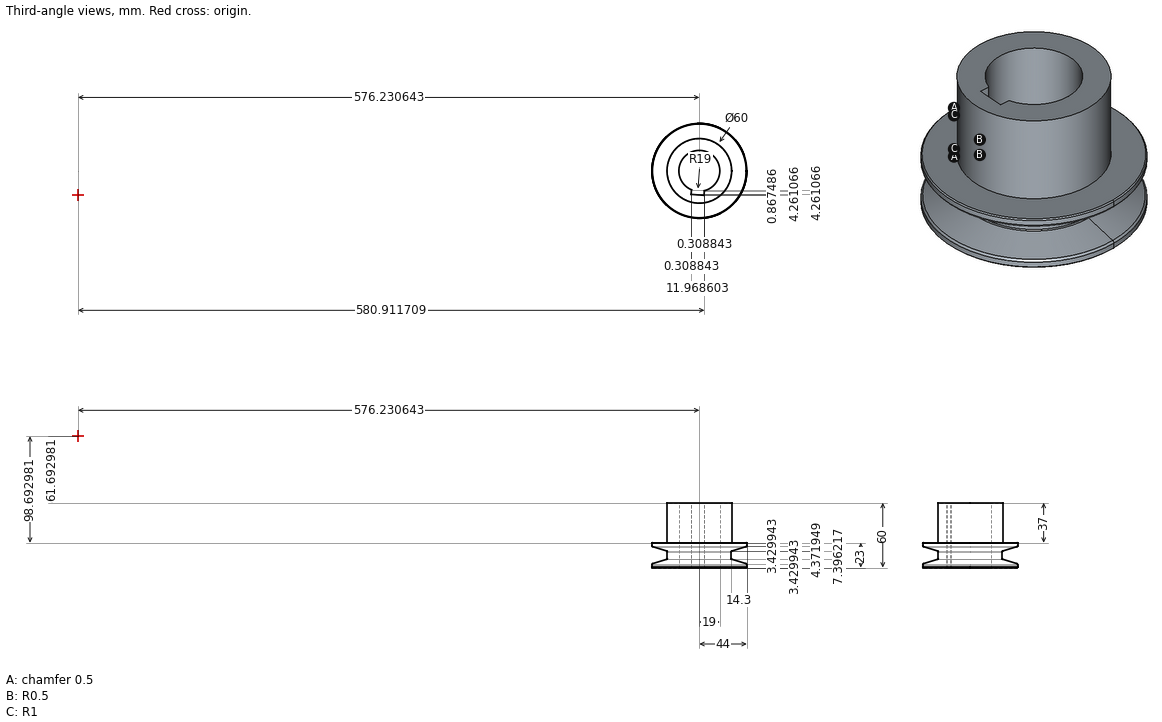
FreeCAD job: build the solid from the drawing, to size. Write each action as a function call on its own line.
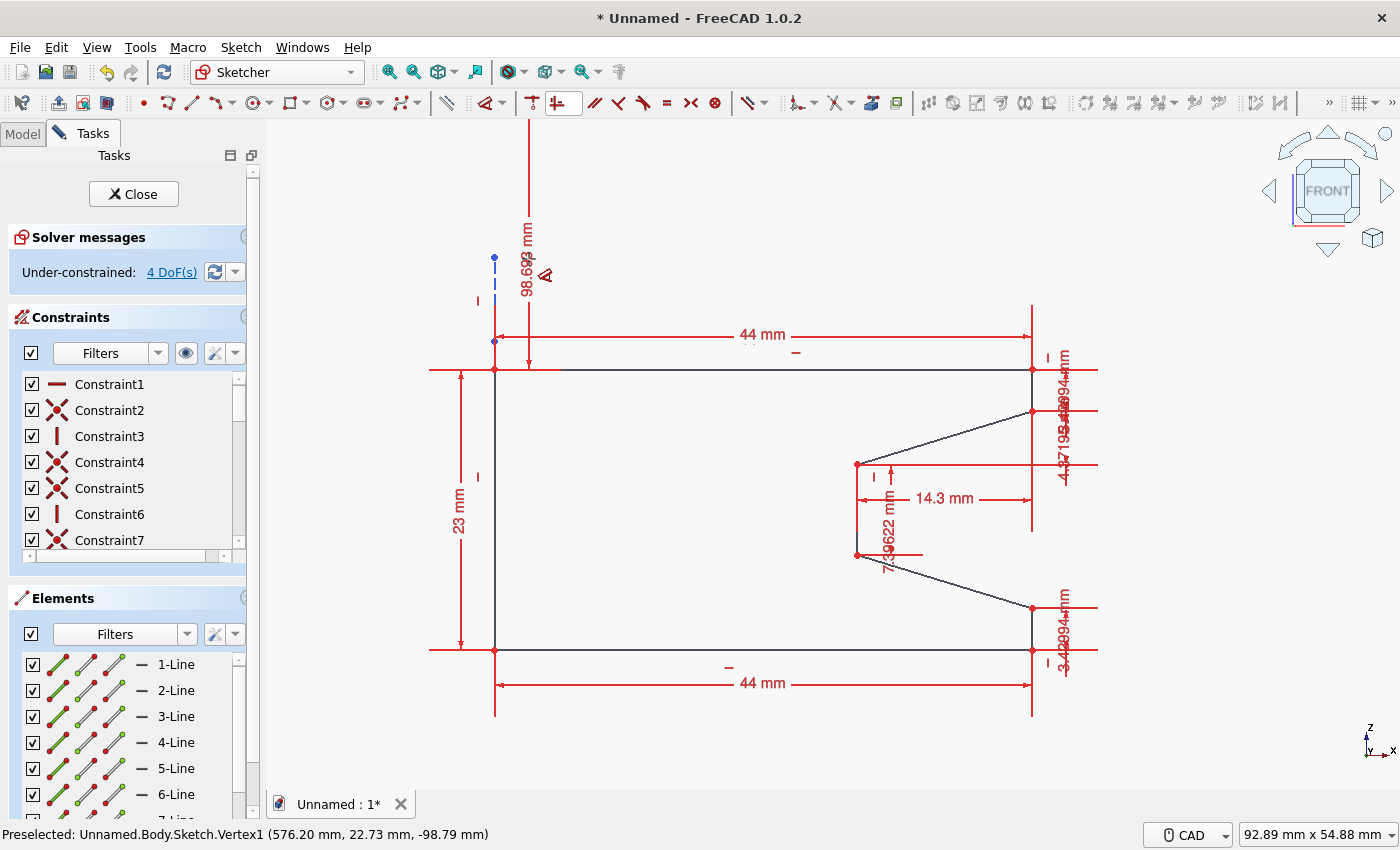
click(495, 370)
click(394, 404)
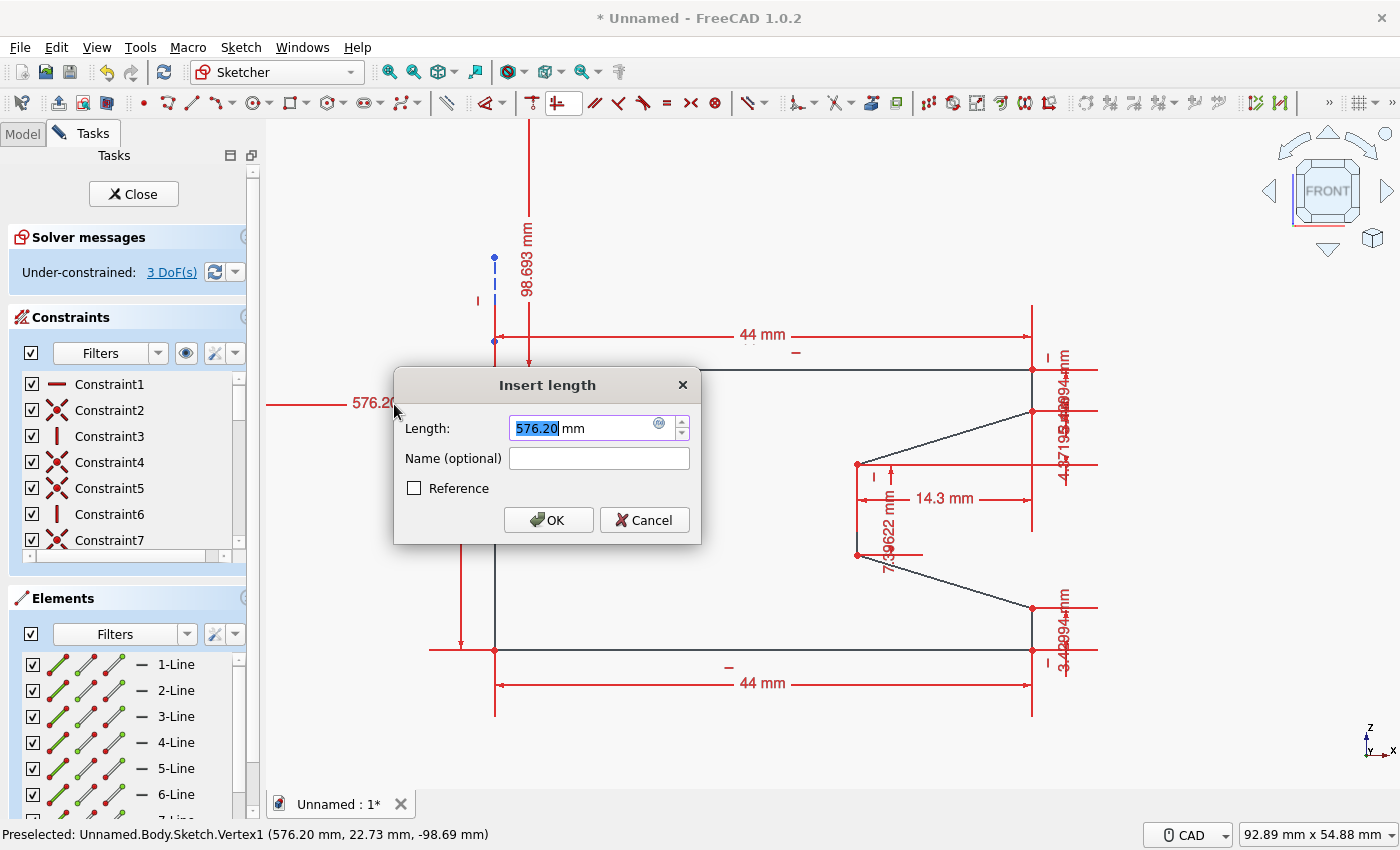
text(576.230643)
key(Return)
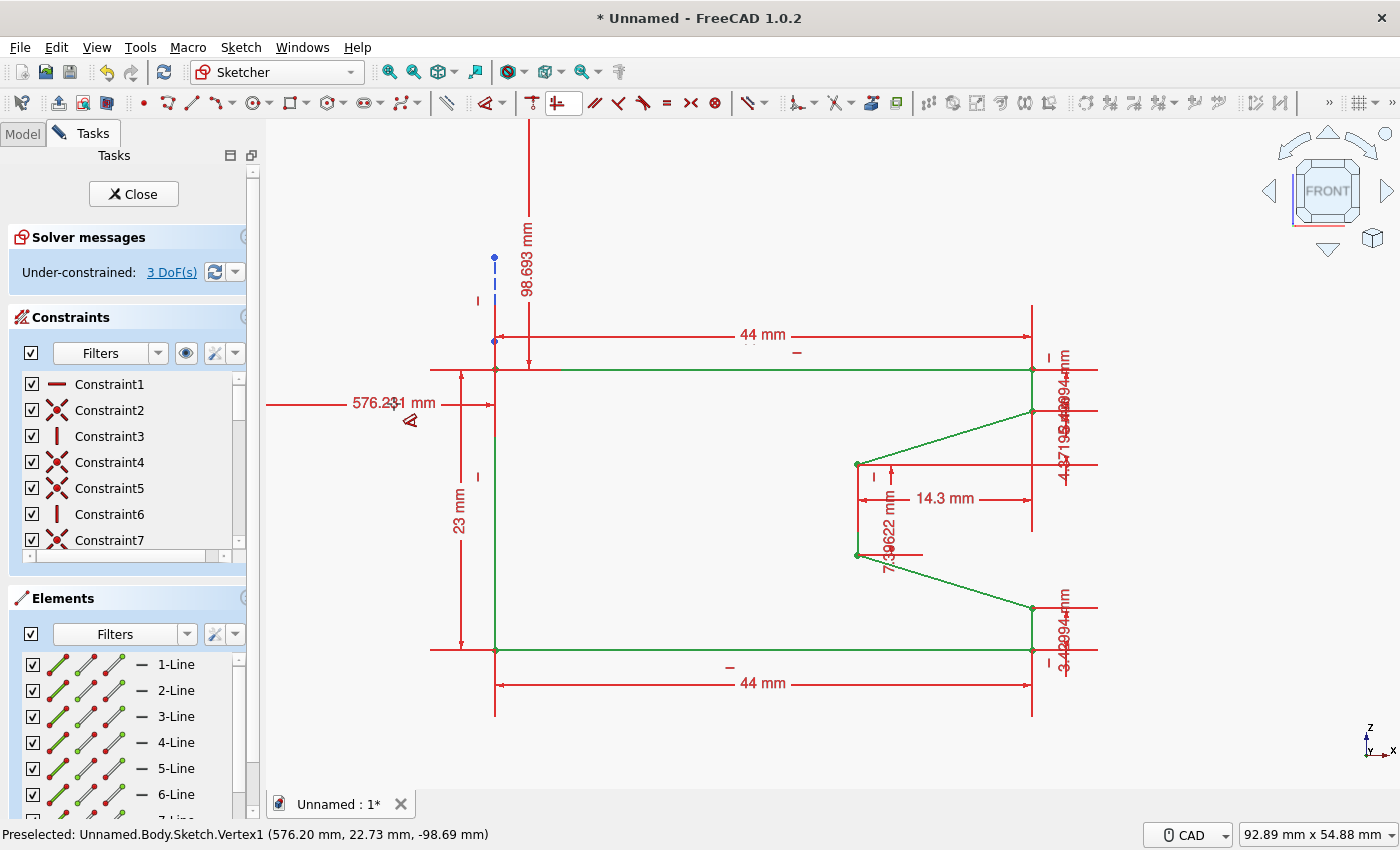
click(495, 342)
click(394, 376)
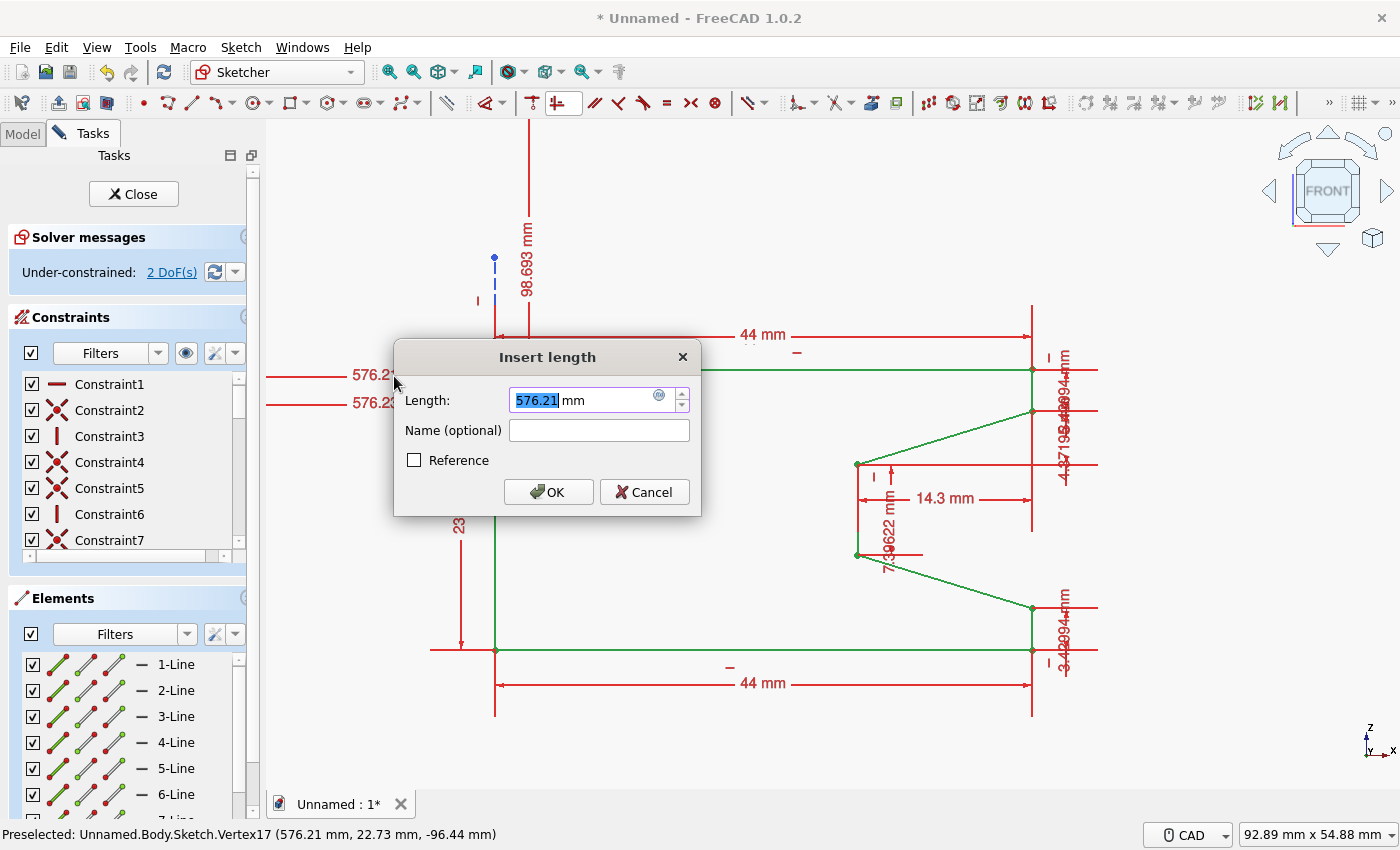
text(576.230643)
key(Return)
key(Escape)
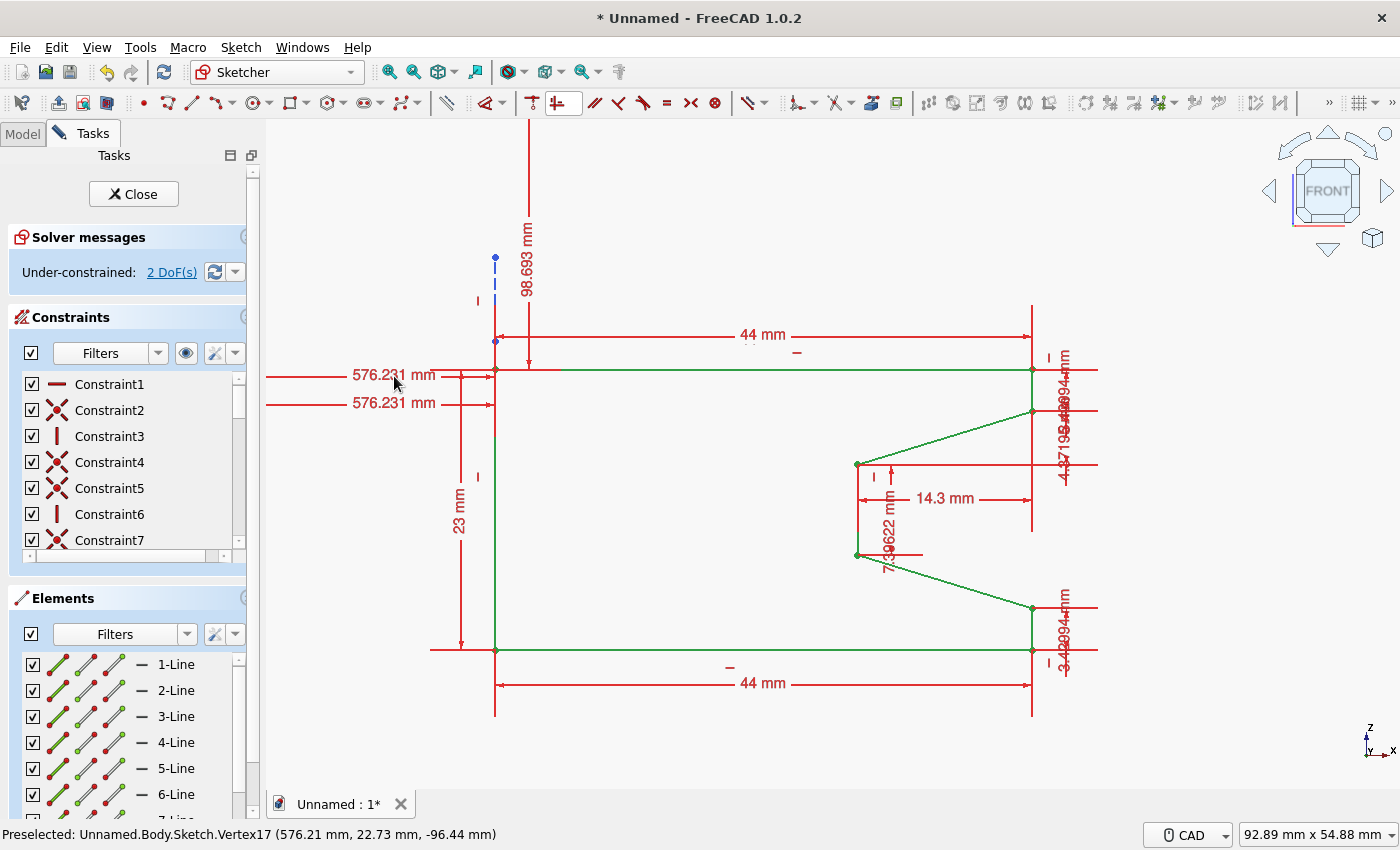
click(134, 194)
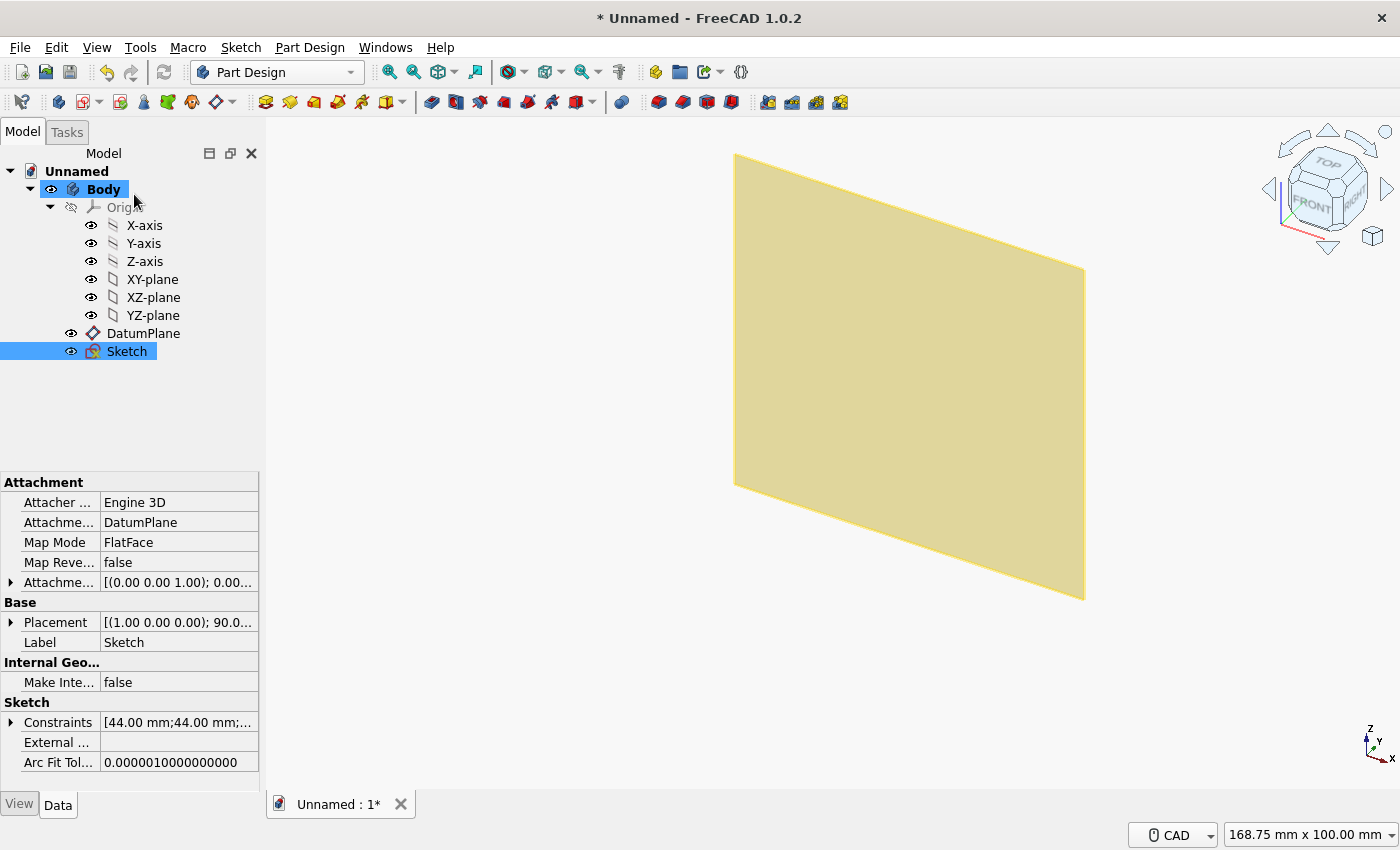
click(290, 102)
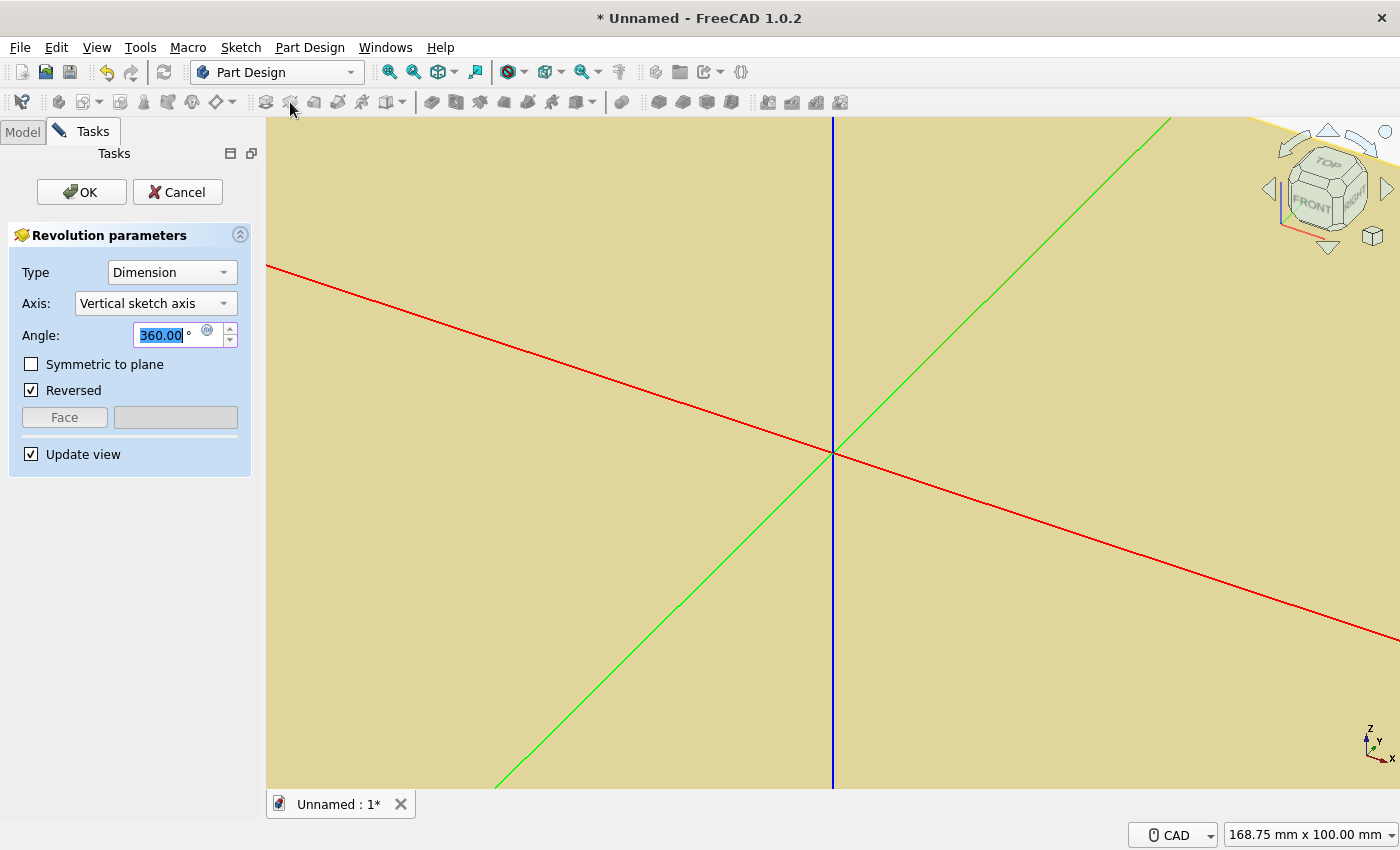
click(156, 304)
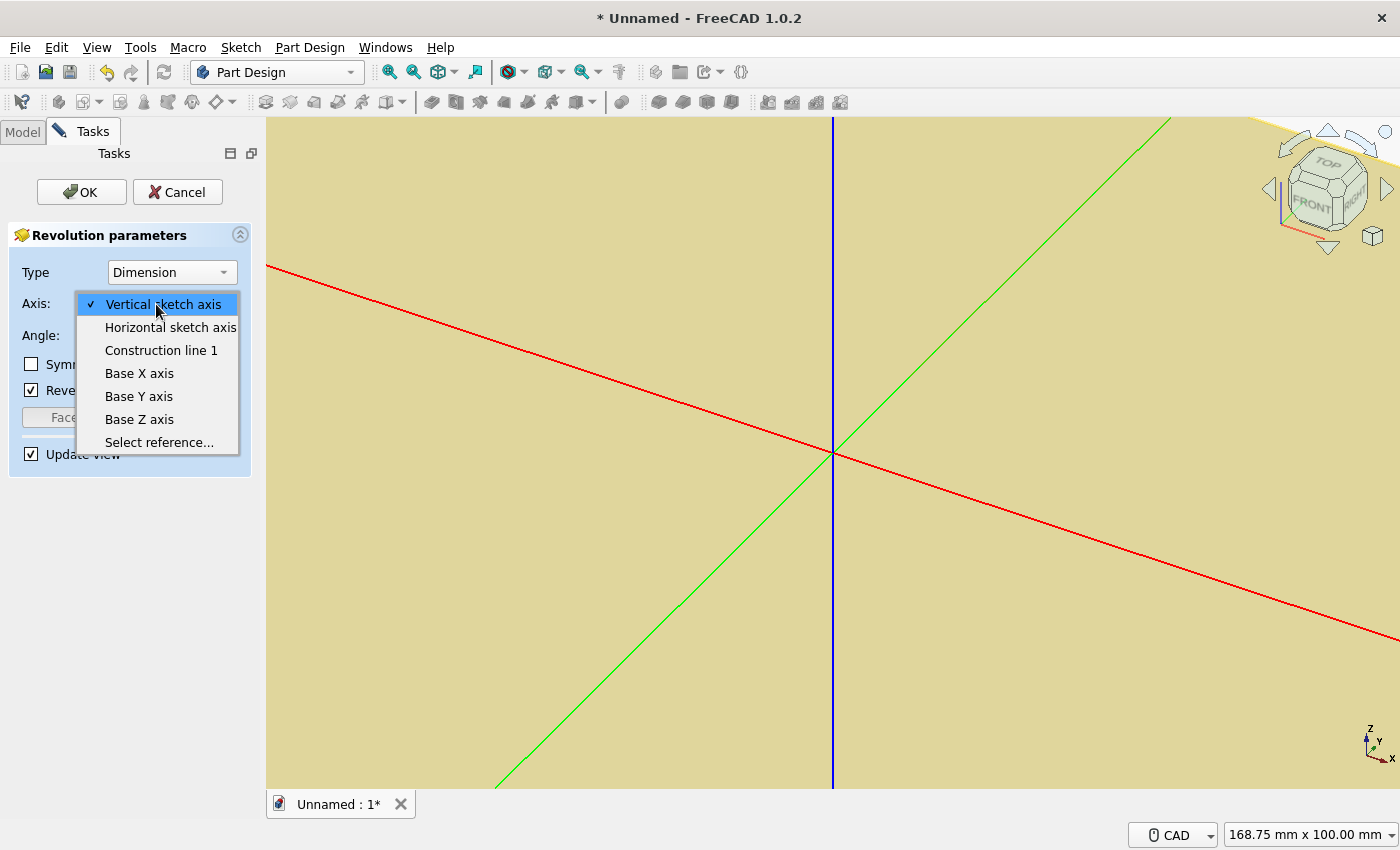
click(156, 350)